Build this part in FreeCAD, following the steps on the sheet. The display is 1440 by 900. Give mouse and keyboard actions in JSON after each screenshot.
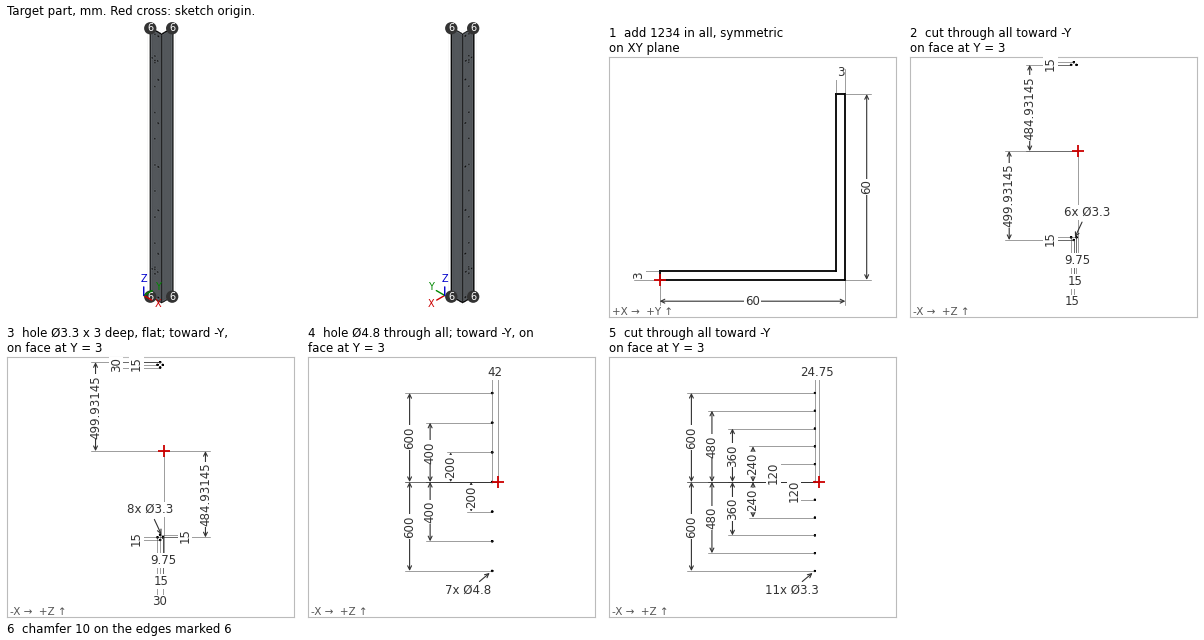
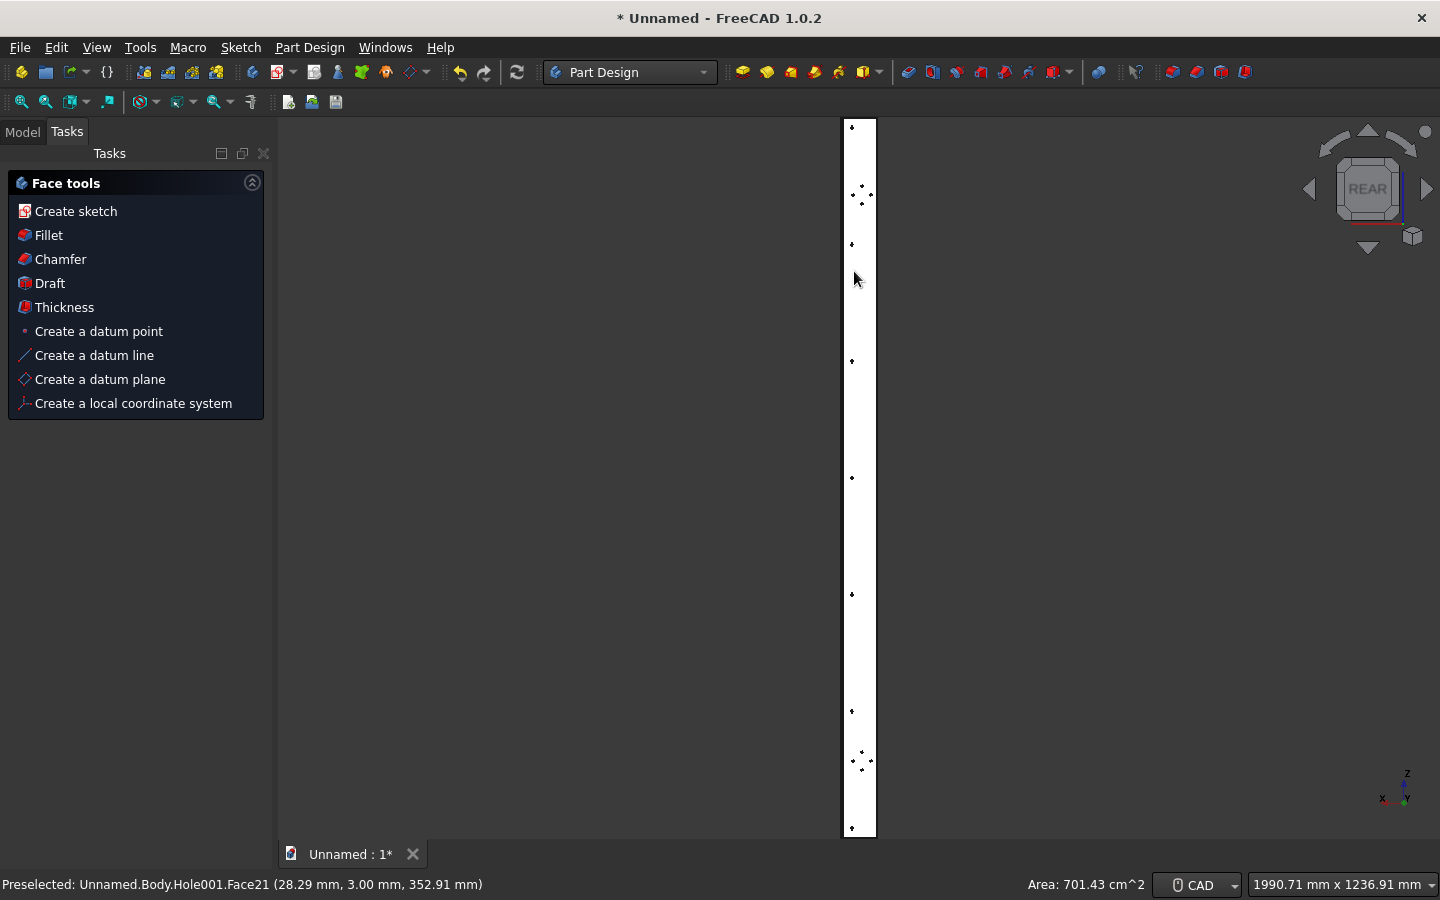
{"action": "left_click", "coordinate": [278, 72]}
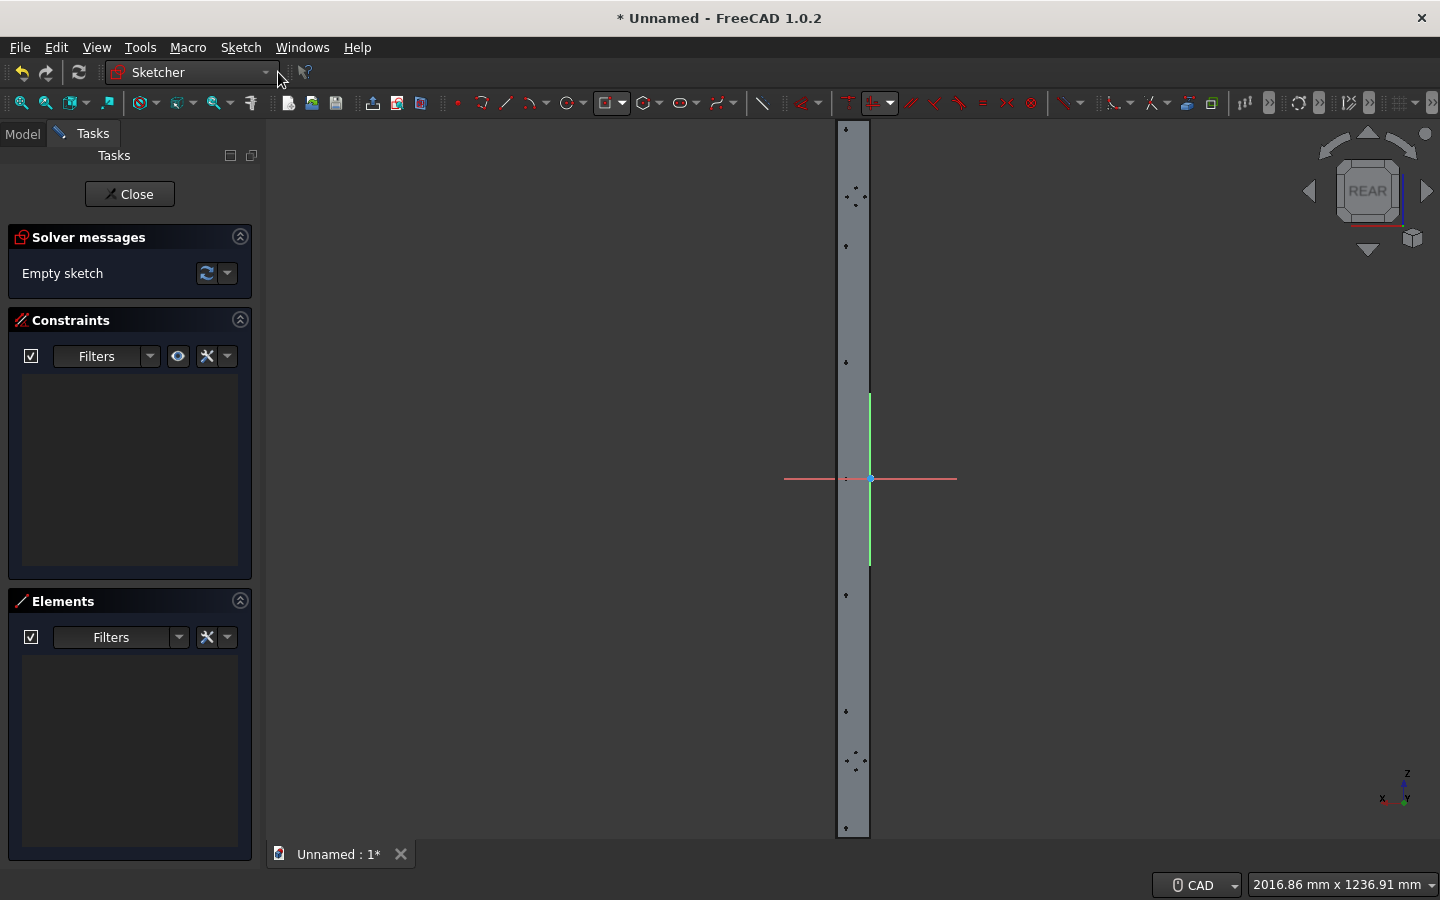
{"action": "scroll", "coordinate": [625, 479], "scroll_direction": "down", "scroll_amount": 2}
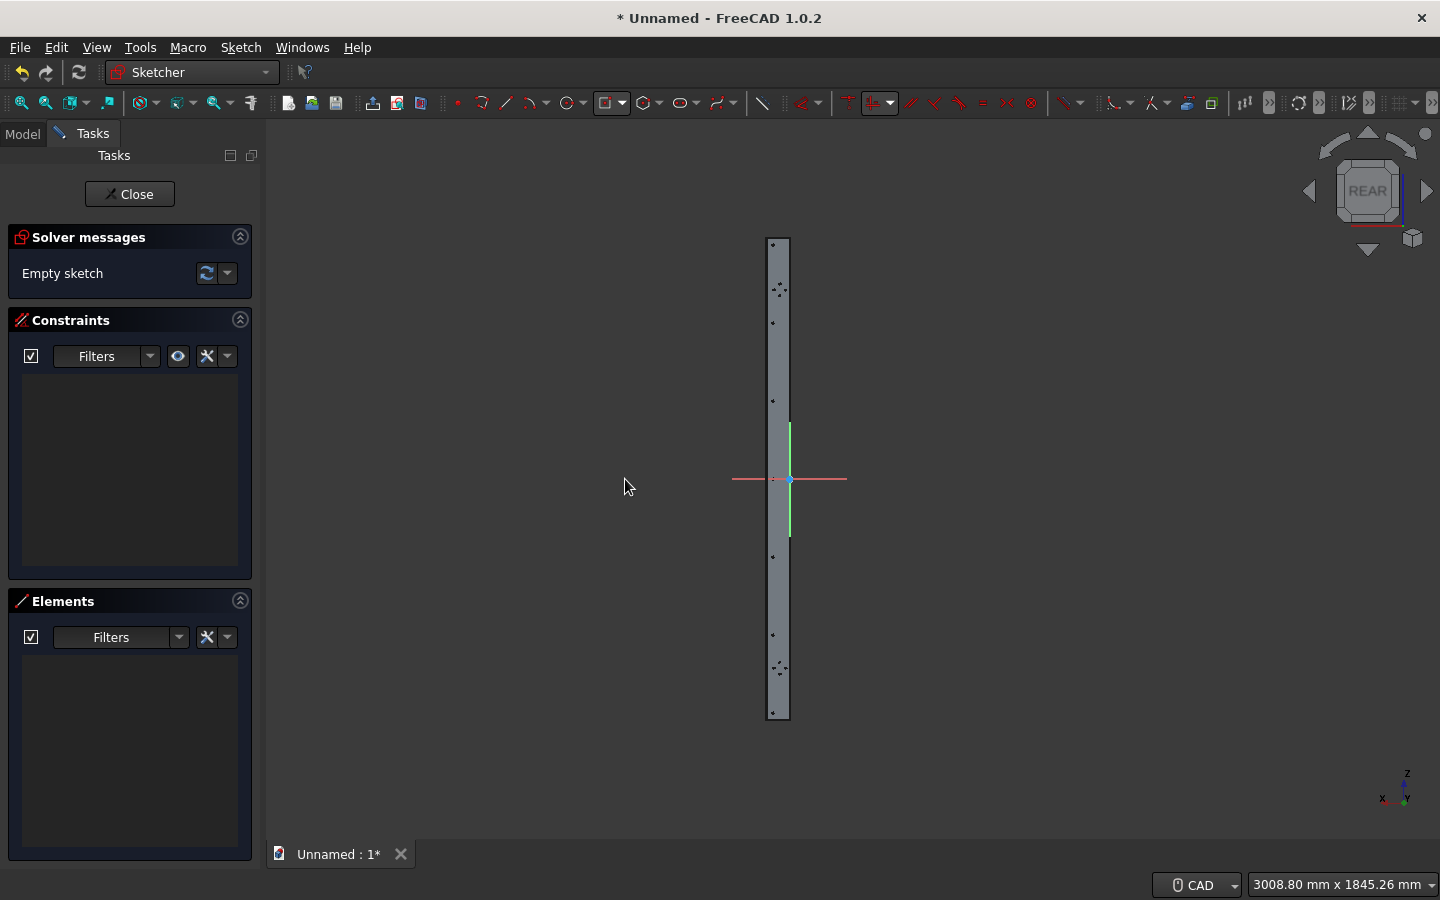
{"action": "left_click", "coordinate": [568, 104]}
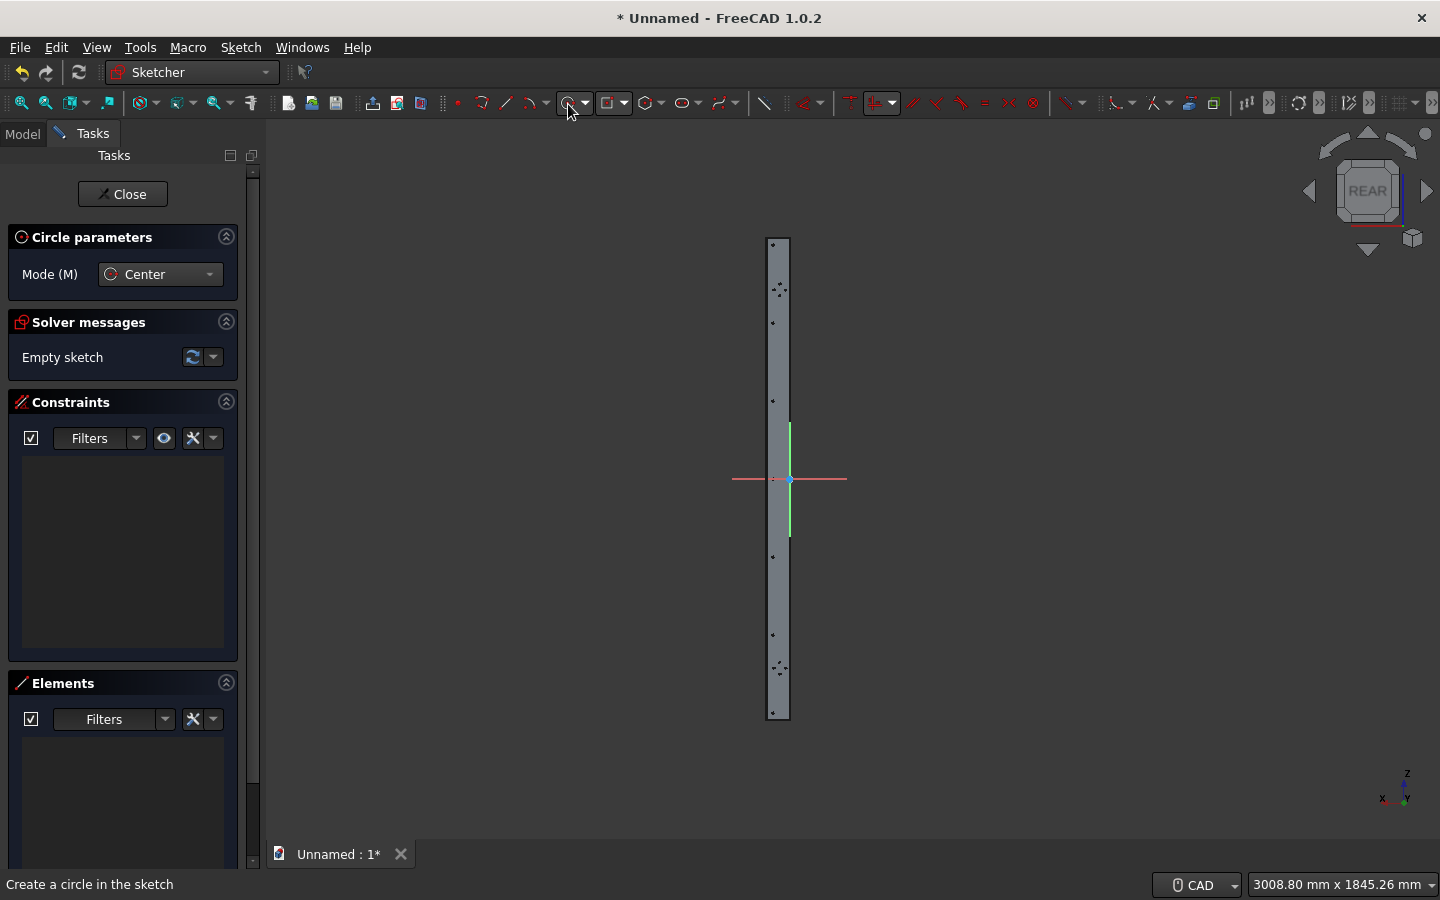
{"action": "scroll", "coordinate": [780, 479], "scroll_direction": "up", "scroll_amount": 18}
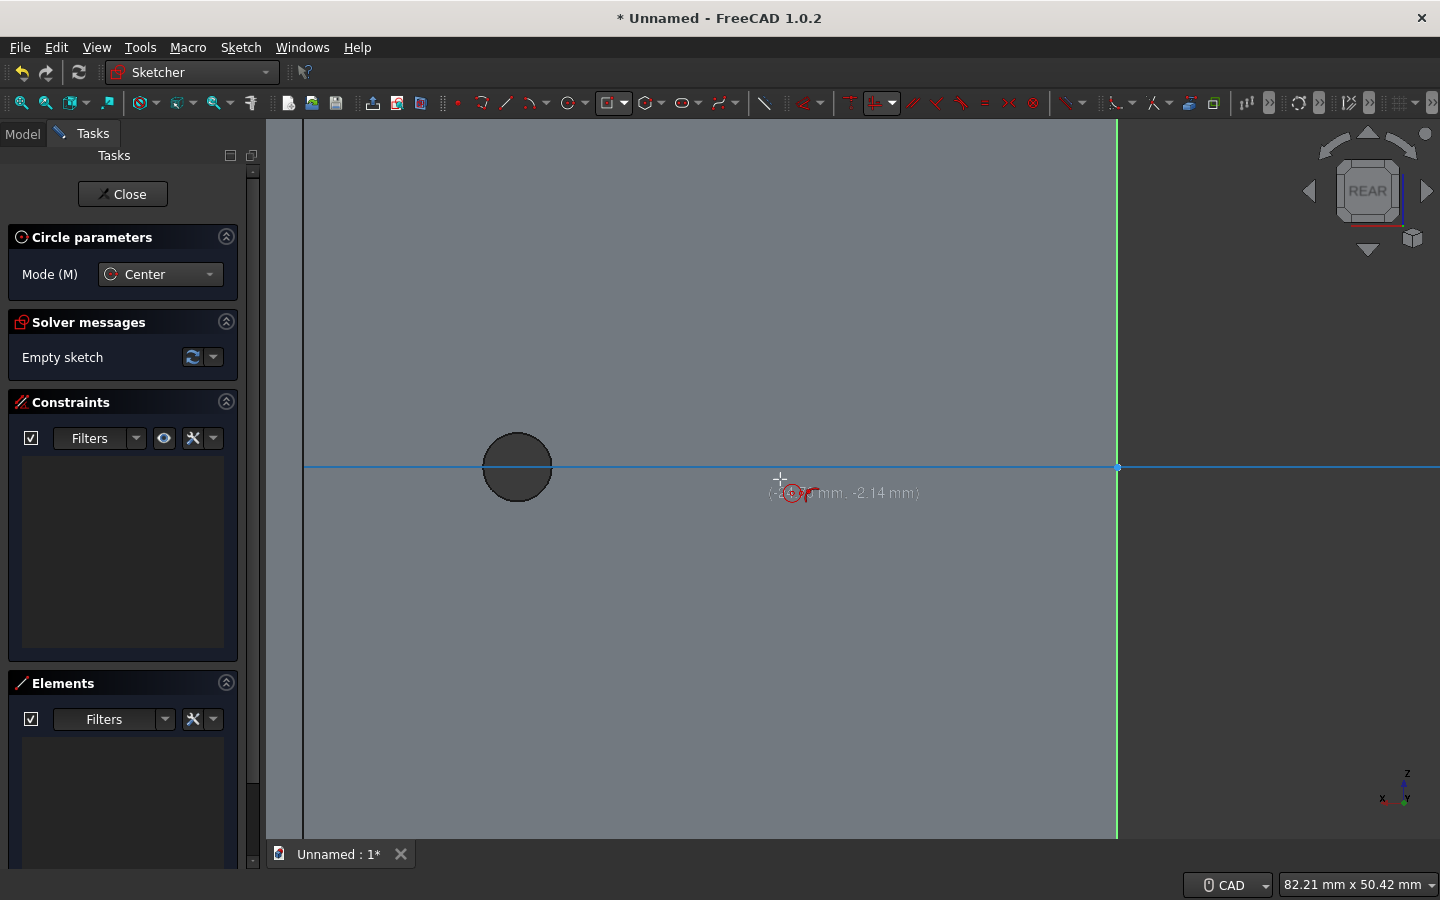
{"action": "scroll", "coordinate": [780, 479], "scroll_direction": "down", "scroll_amount": 17}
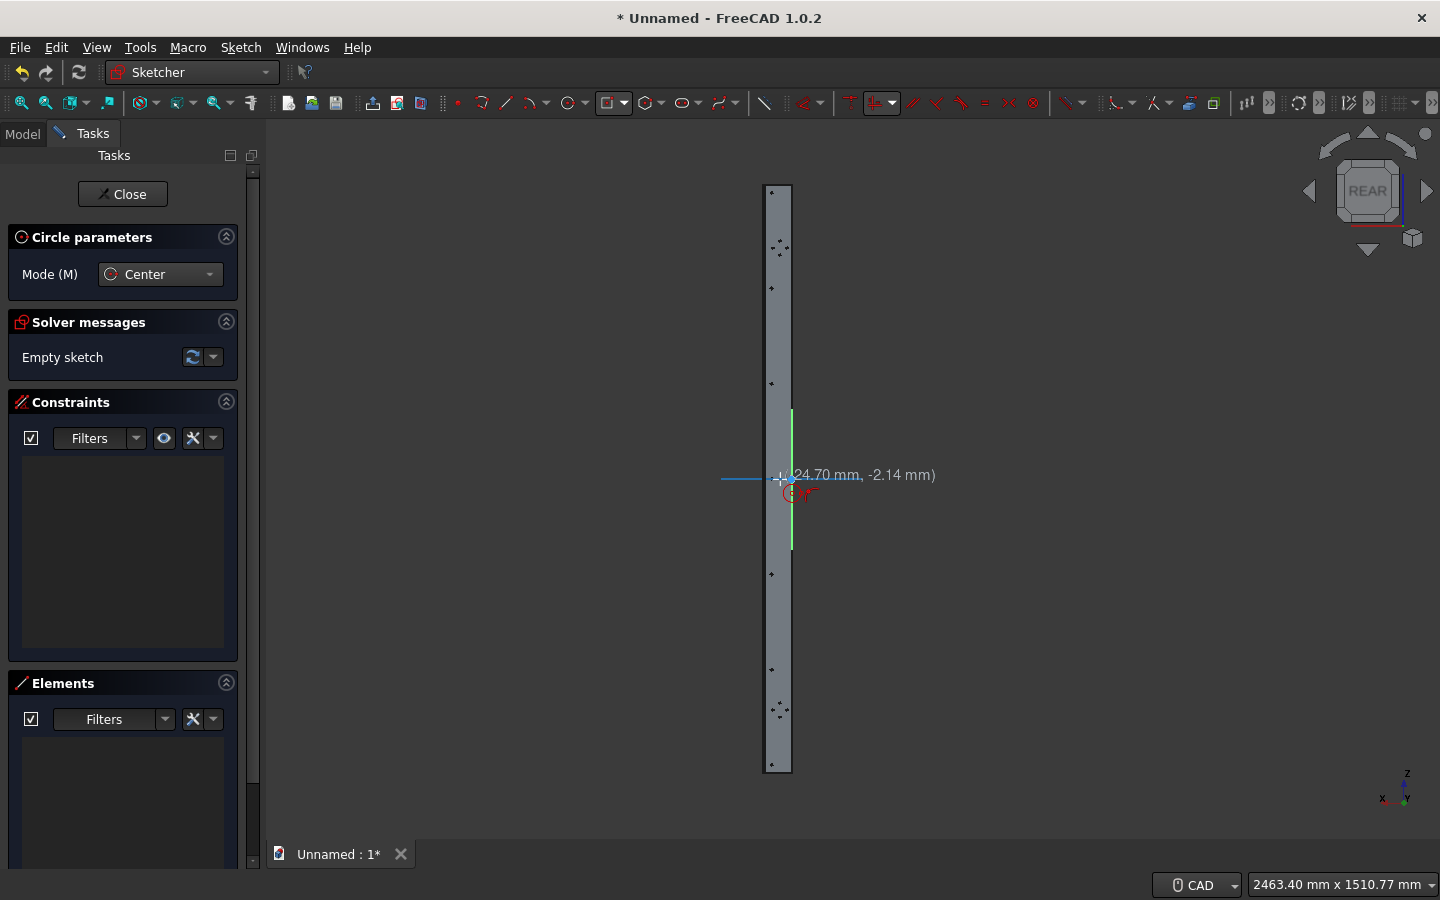
{"action": "scroll", "coordinate": [780, 479], "scroll_direction": "up", "scroll_amount": 2}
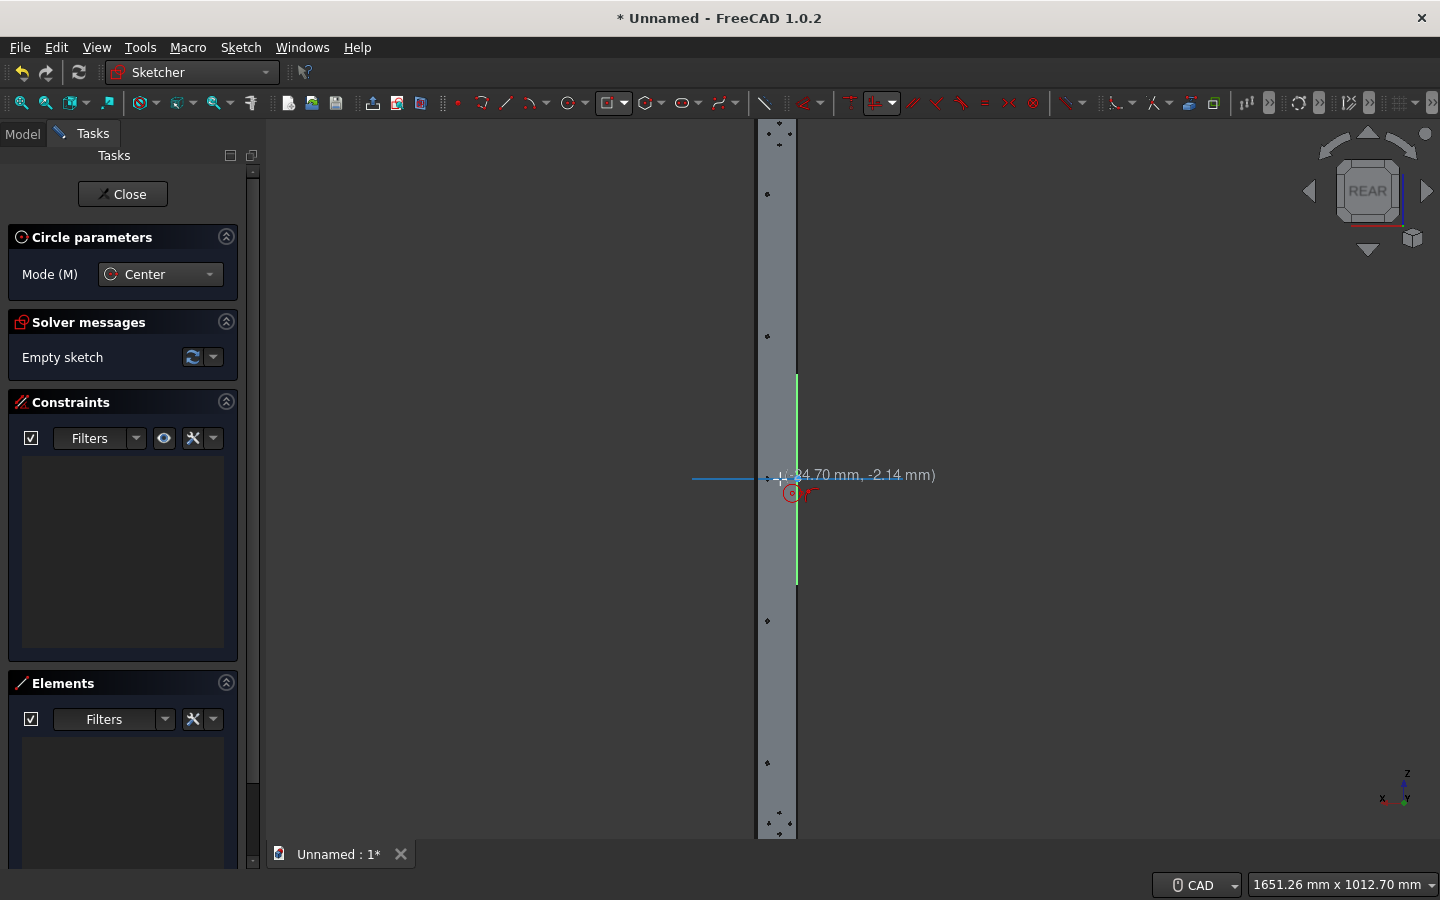
{"action": "left_click", "coordinate": [780, 479]}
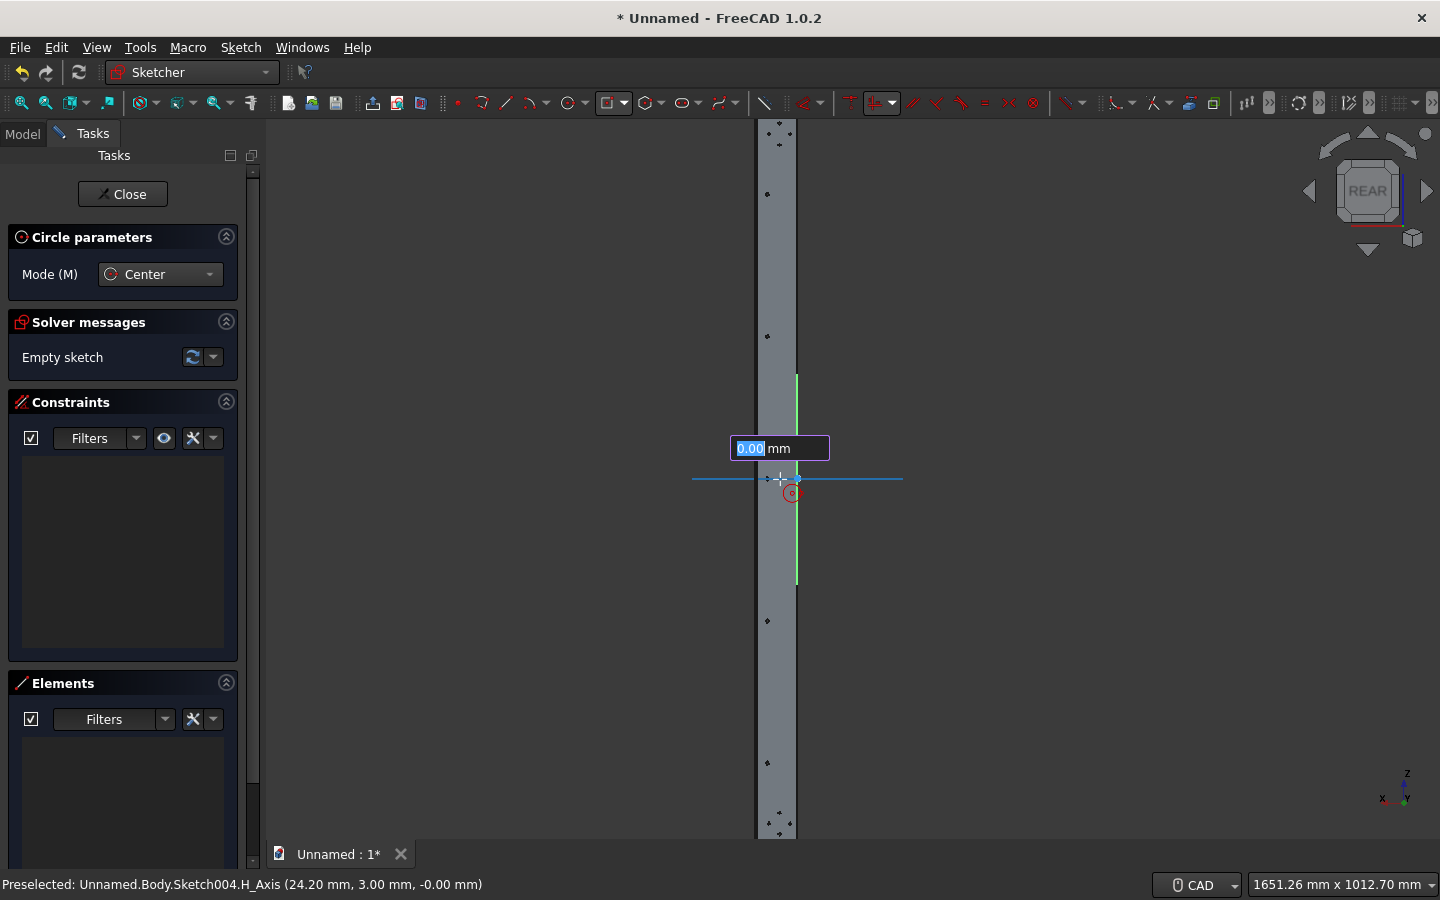
{"action": "scroll", "coordinate": [779, 480], "scroll_direction": "up", "scroll_amount": 14}
{"action": "mouse_move", "coordinate": [776, 472]}